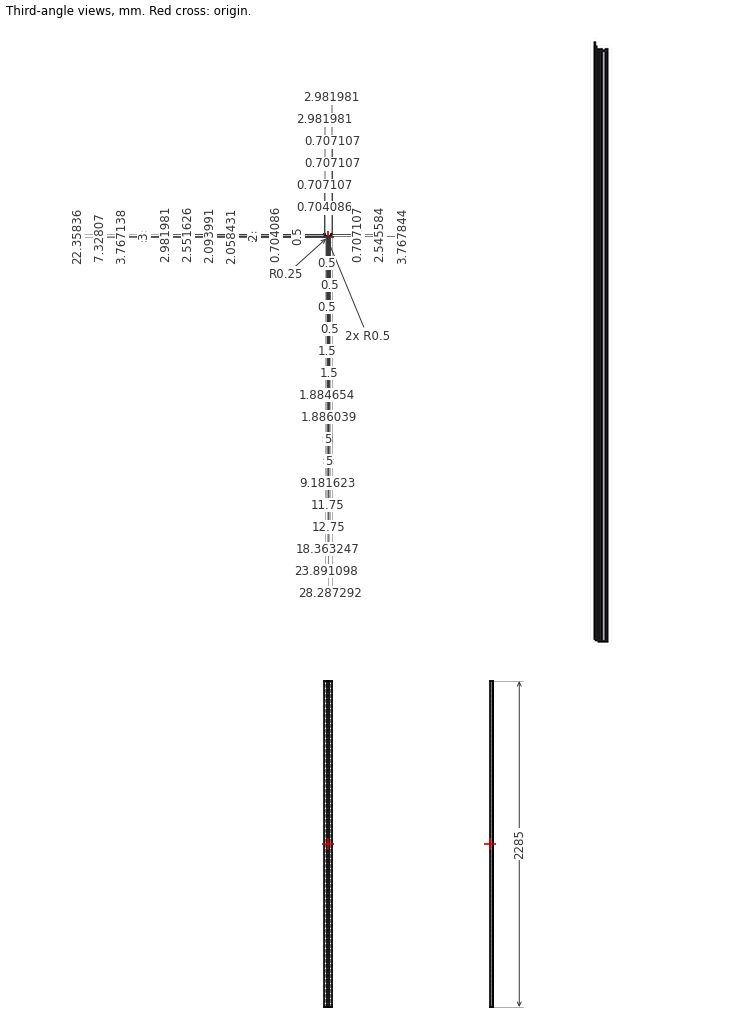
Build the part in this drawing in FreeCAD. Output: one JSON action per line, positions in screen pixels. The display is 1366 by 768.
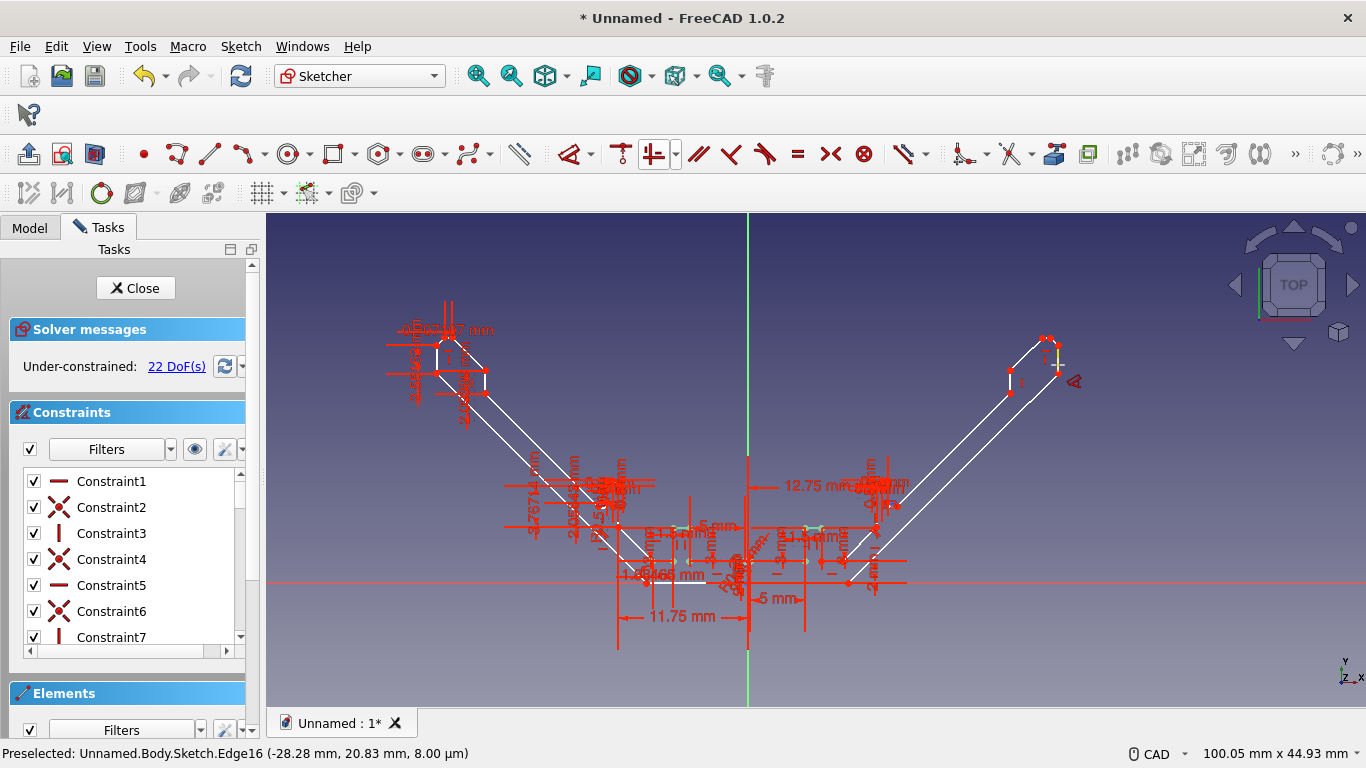
{"action": "left_click", "coordinate": [1058, 365]}
{"action": "left_click", "coordinate": [1092, 355]}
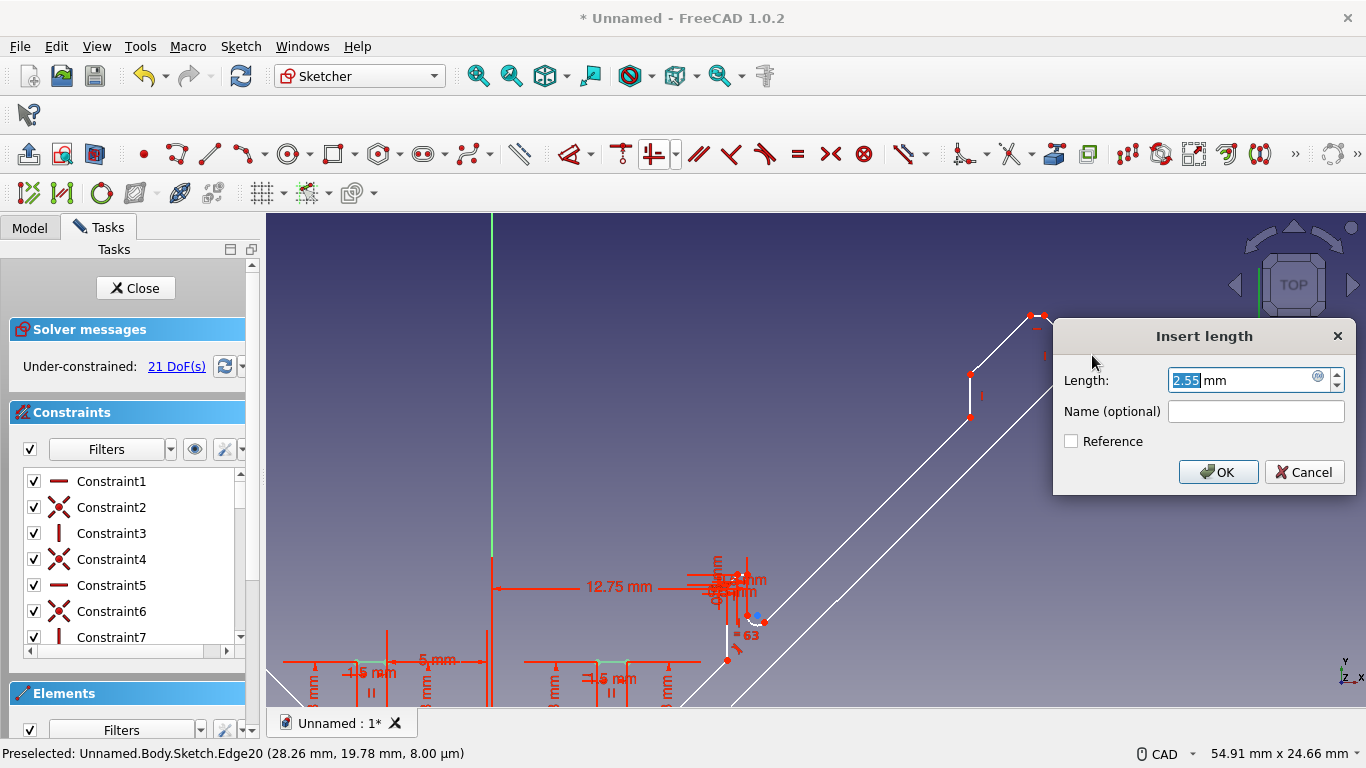
{"action": "type", "text": "2.545584"}
{"action": "key", "text": "Return"}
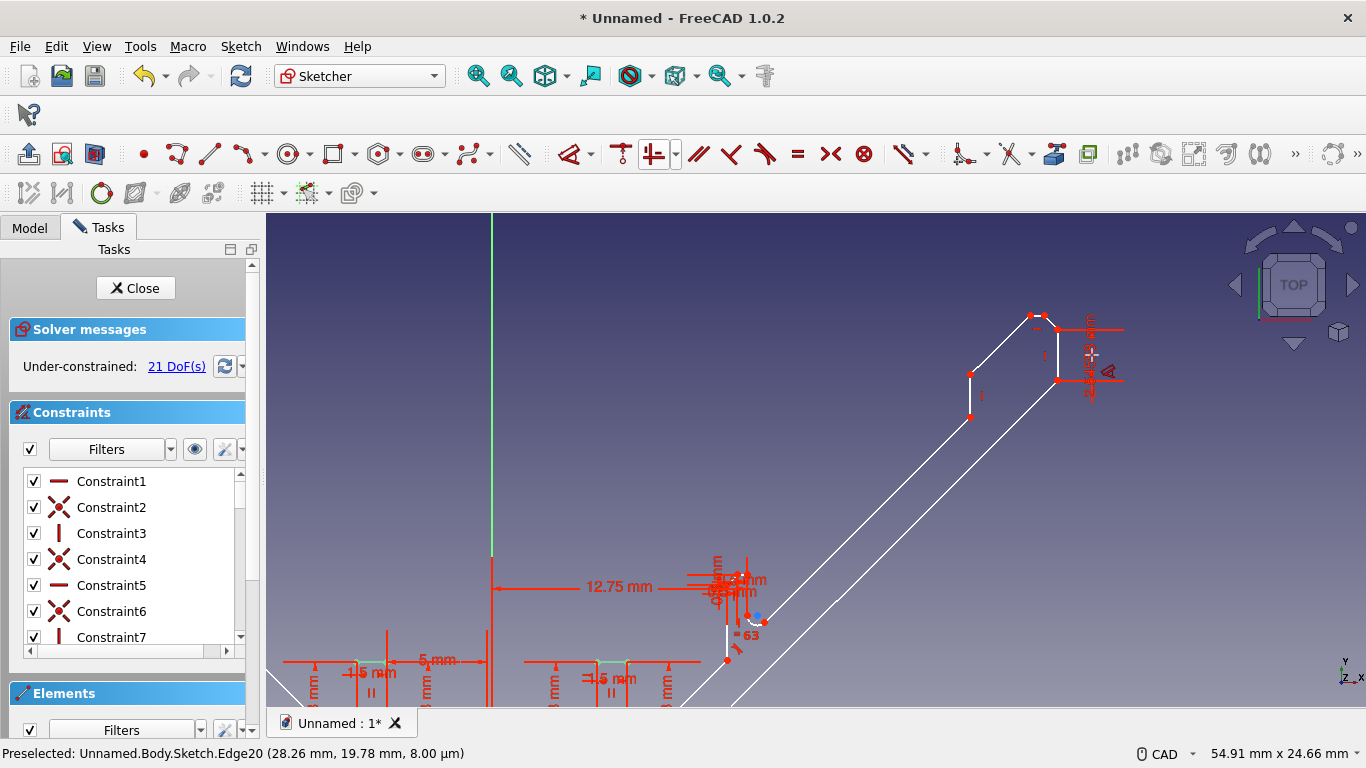
{"action": "scroll", "coordinate": [1037, 316], "scroll_direction": "up", "scroll_amount": 6}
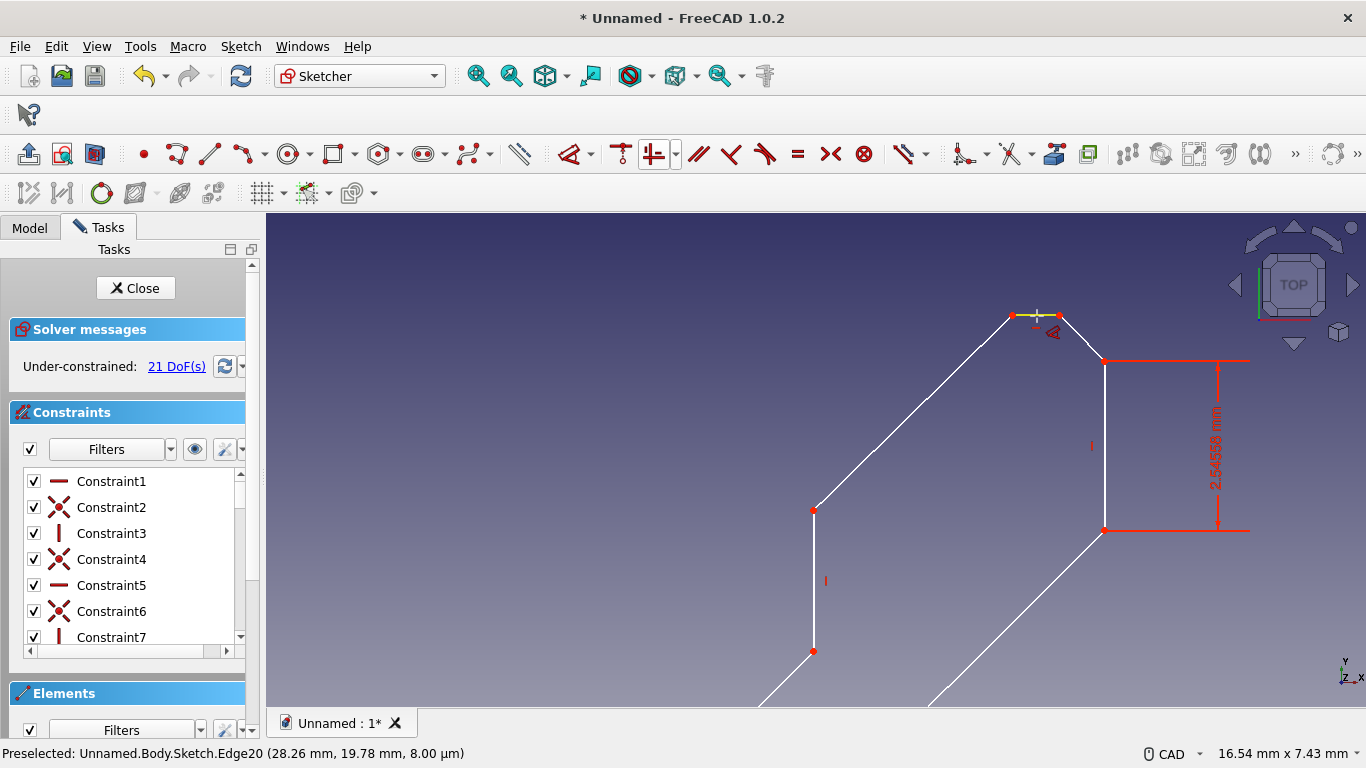
{"action": "left_click", "coordinate": [1036, 315]}
{"action": "left_click", "coordinate": [1036, 281]}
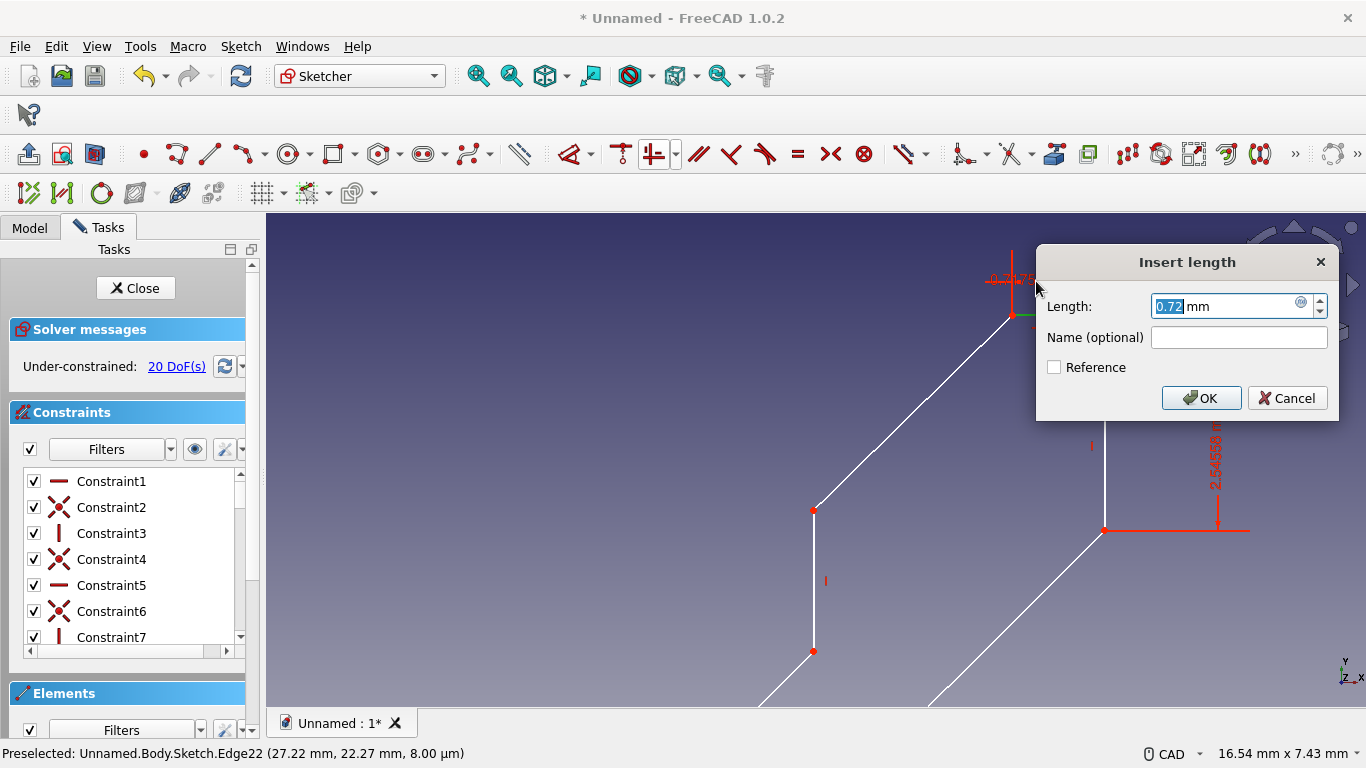
{"action": "type", "text": "0.707107"}
{"action": "key", "text": "Return"}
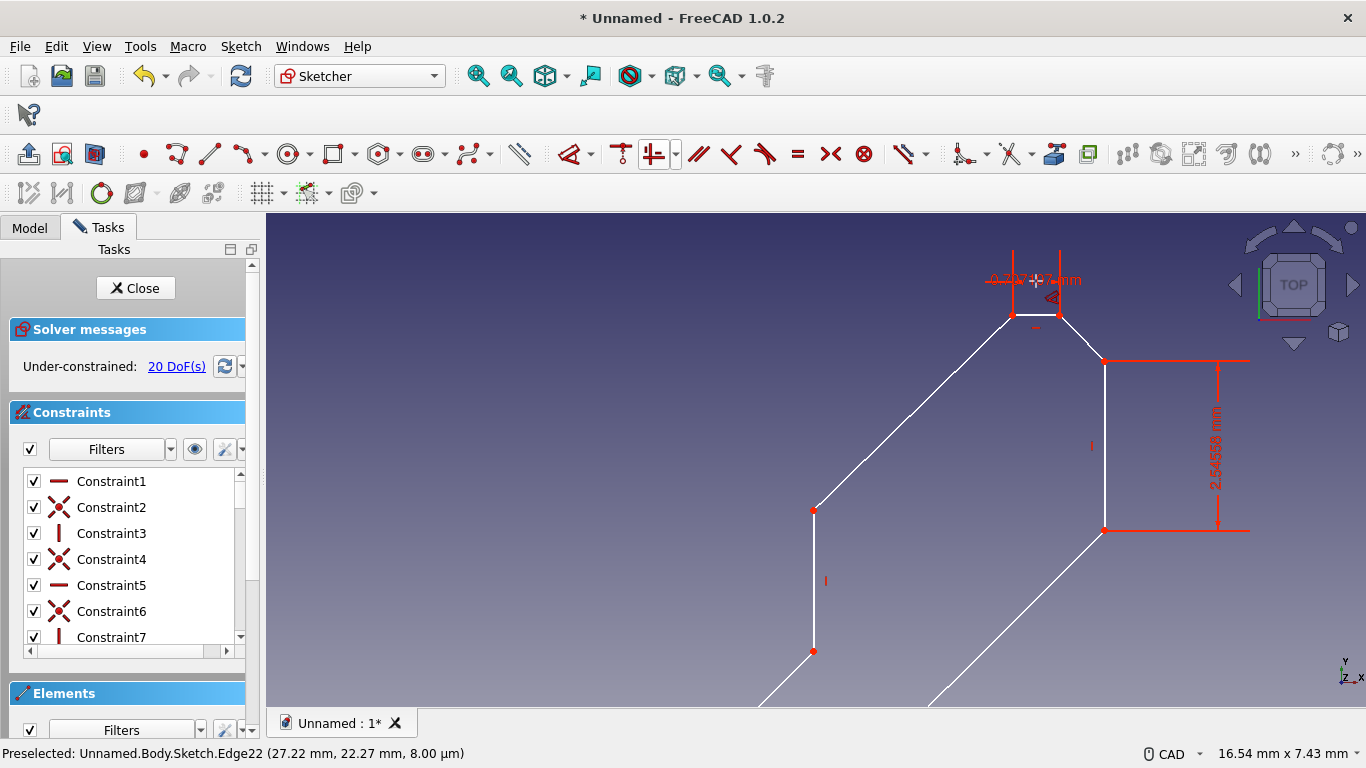
{"action": "scroll", "coordinate": [1049, 343], "scroll_direction": "down", "scroll_amount": 9}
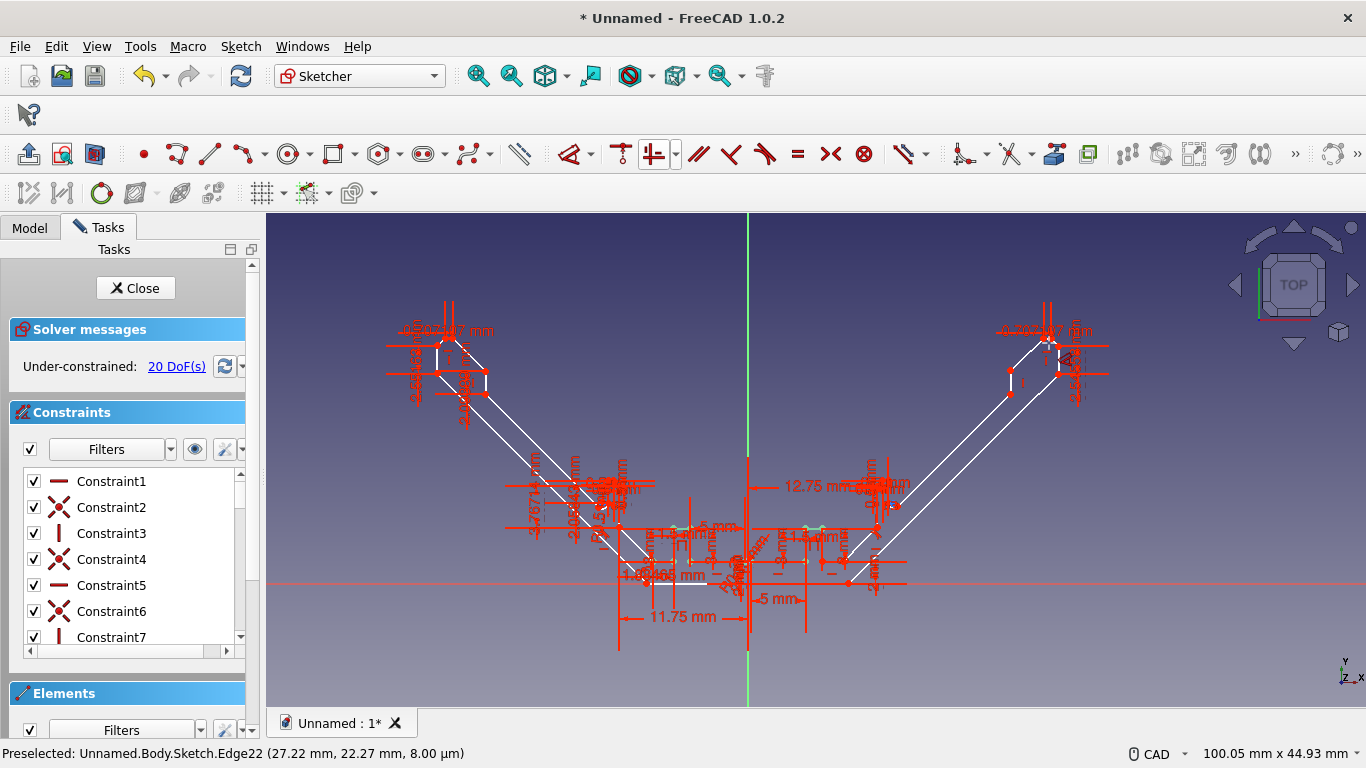
{"action": "scroll", "coordinate": [1011, 378], "scroll_direction": "up", "scroll_amount": 4}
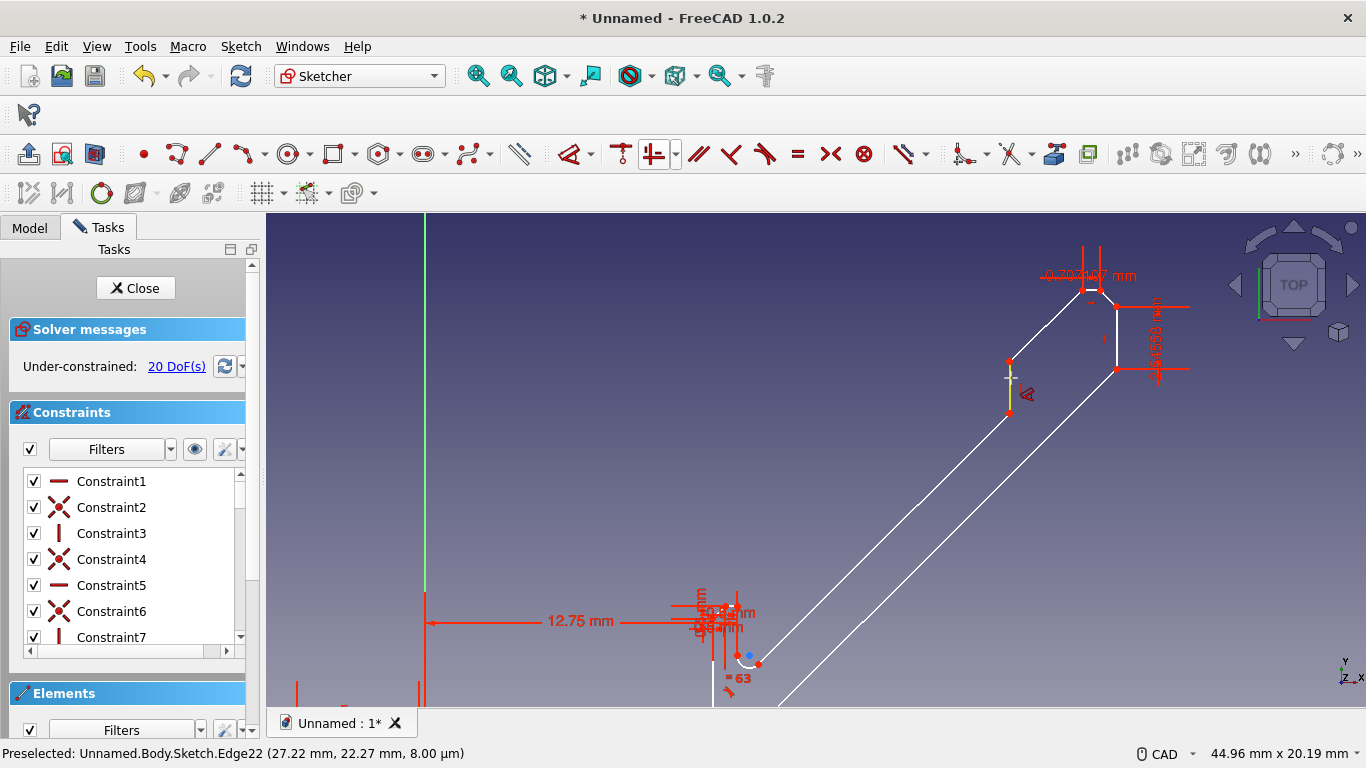
{"action": "left_click", "coordinate": [1010, 377]}
{"action": "left_click", "coordinate": [1044, 388]}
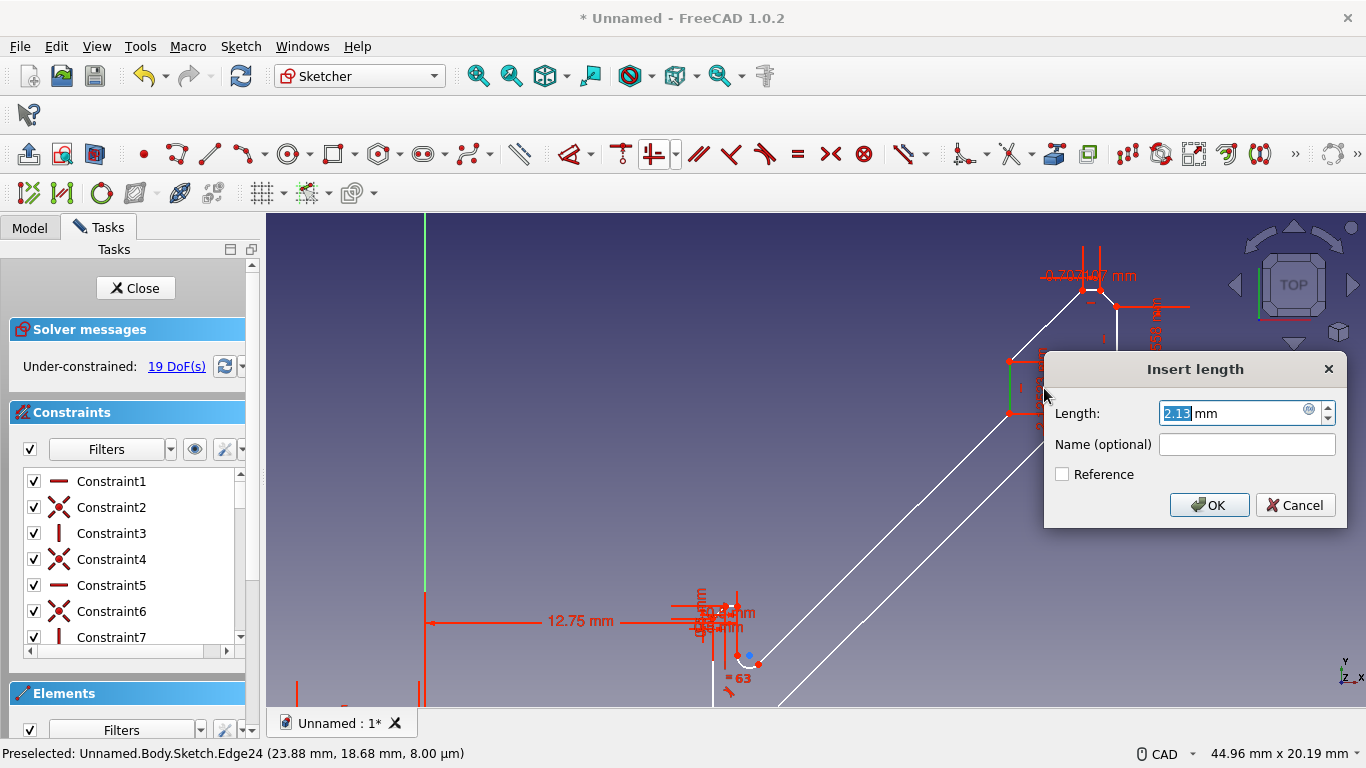
{"action": "type", "text": "2.093991"}
{"action": "key", "text": "Return"}